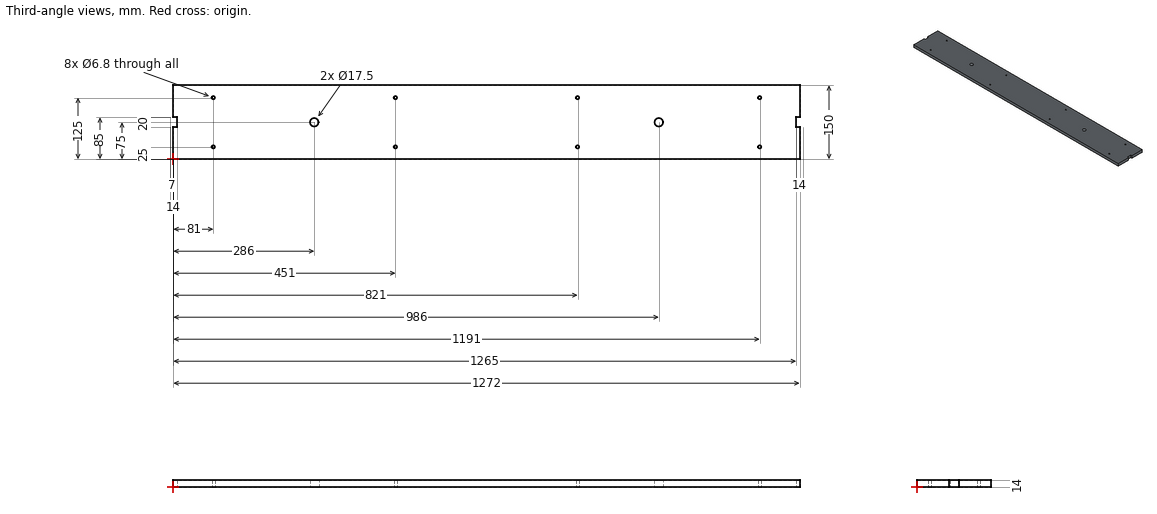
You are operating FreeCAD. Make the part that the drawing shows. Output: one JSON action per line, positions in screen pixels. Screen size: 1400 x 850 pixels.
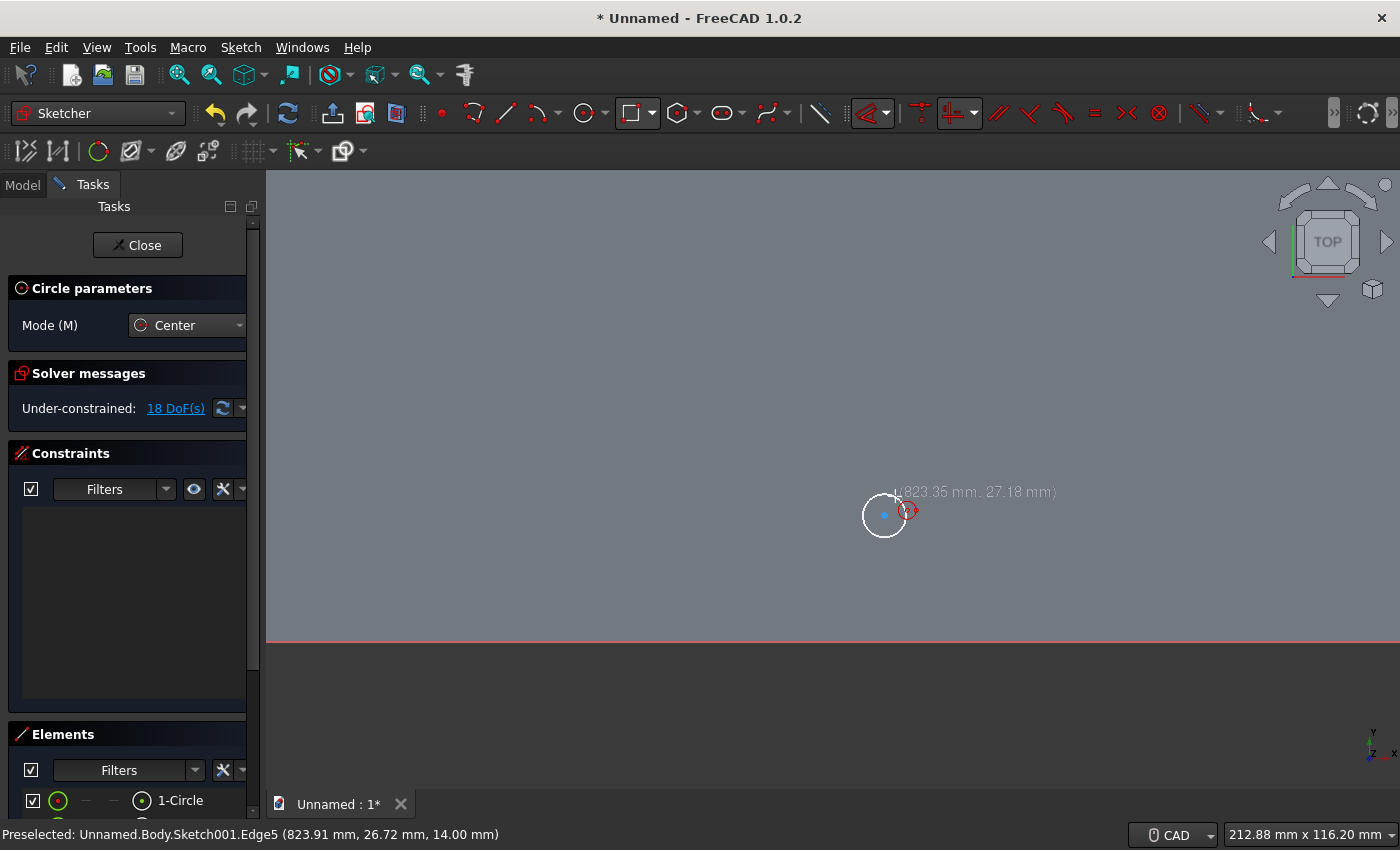
{"action": "scroll", "coordinate": [898, 502], "scroll_direction": "down", "scroll_amount": 11}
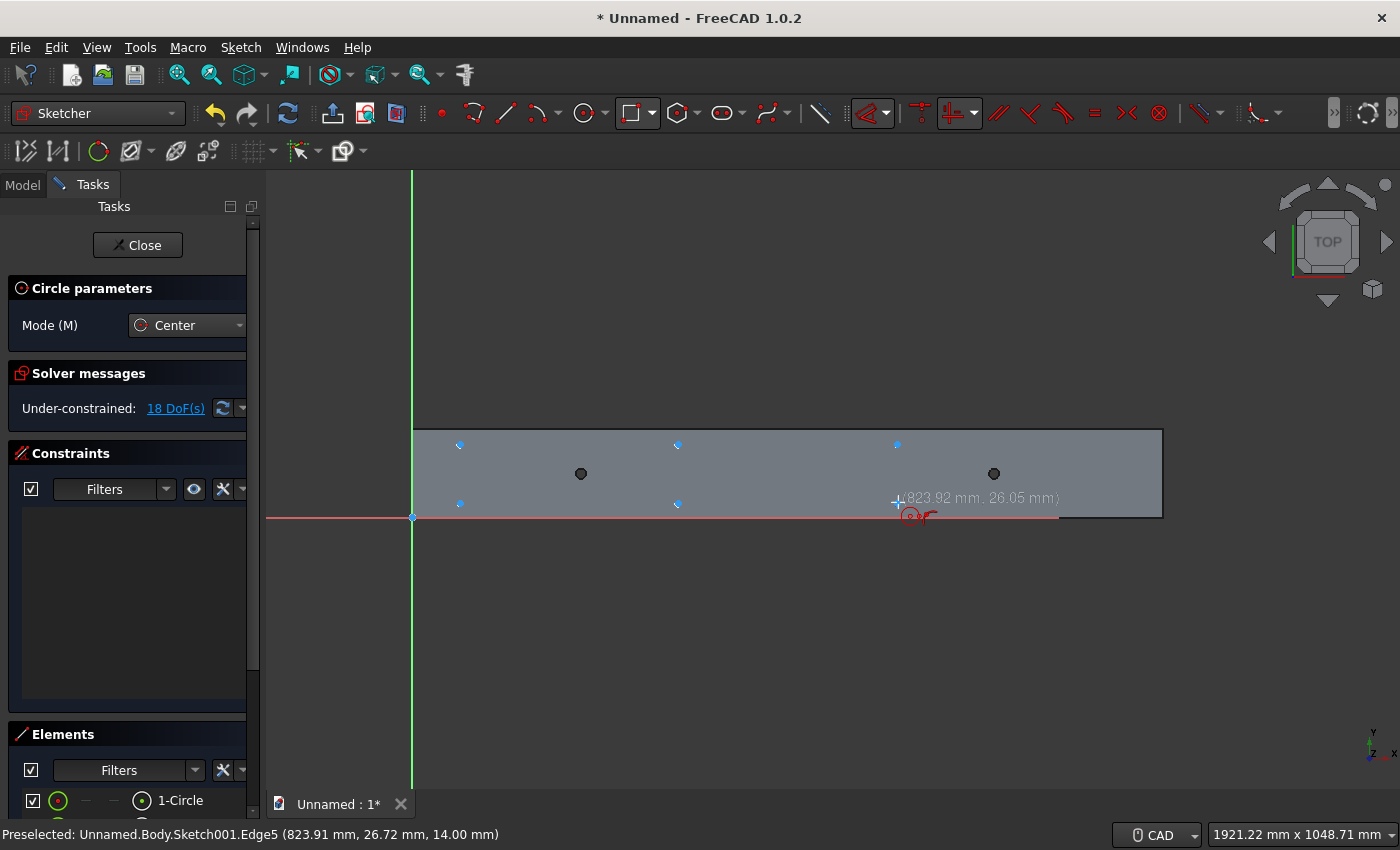
{"action": "scroll", "coordinate": [1115, 444], "scroll_direction": "up", "scroll_amount": 13}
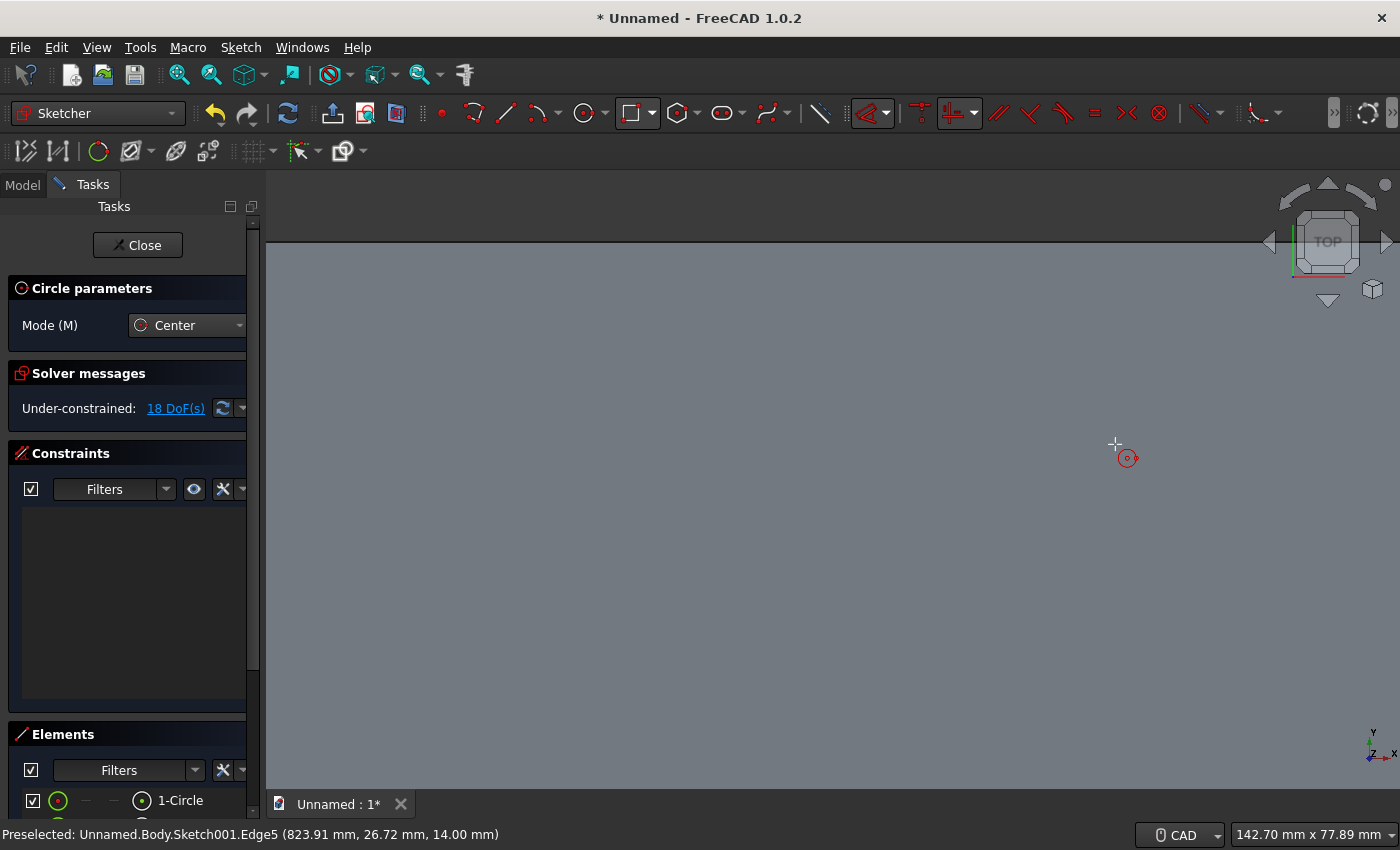
{"action": "scroll", "coordinate": [1116, 444], "scroll_direction": "down", "scroll_amount": 13}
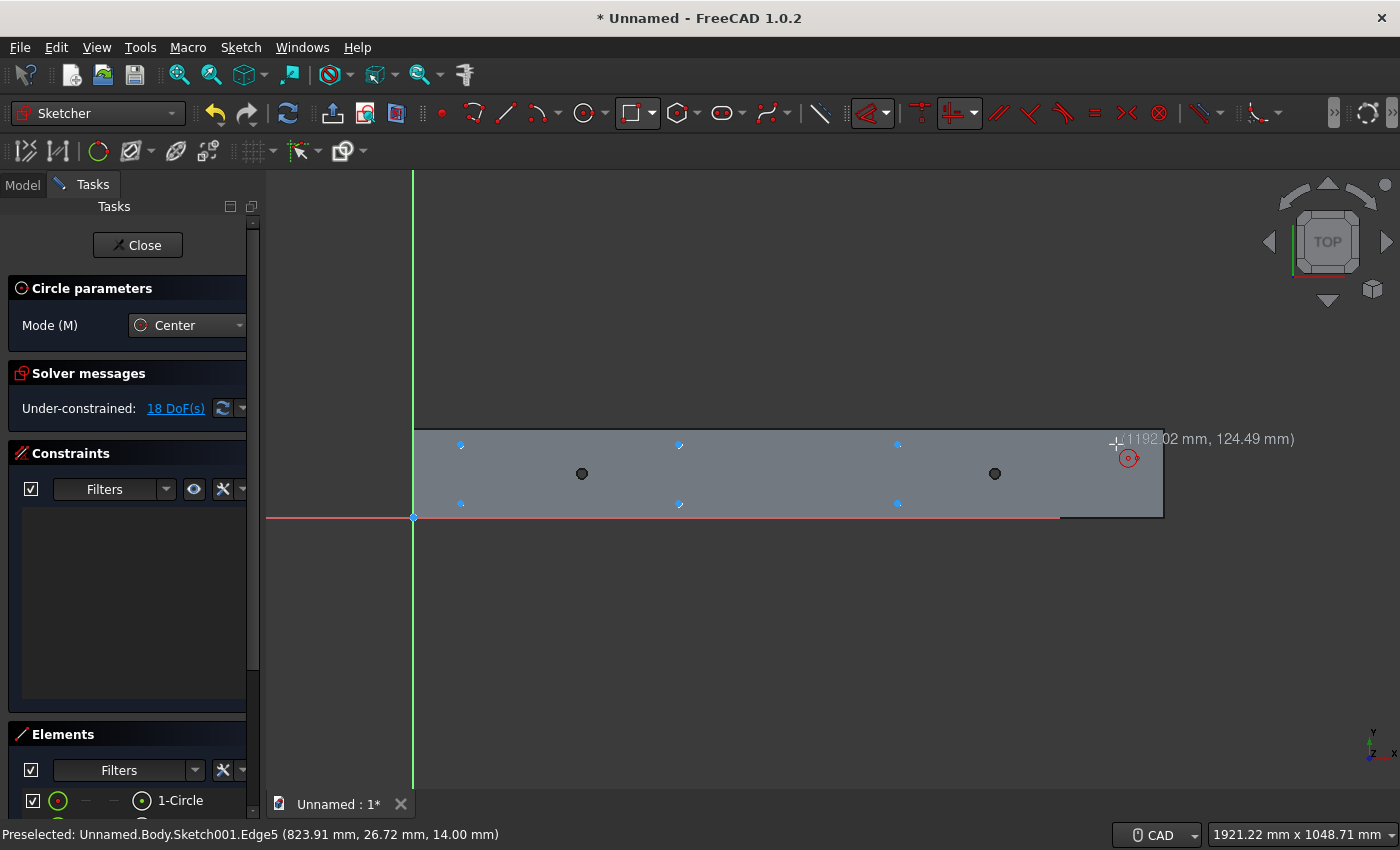
{"action": "left_click", "coordinate": [1116, 444]}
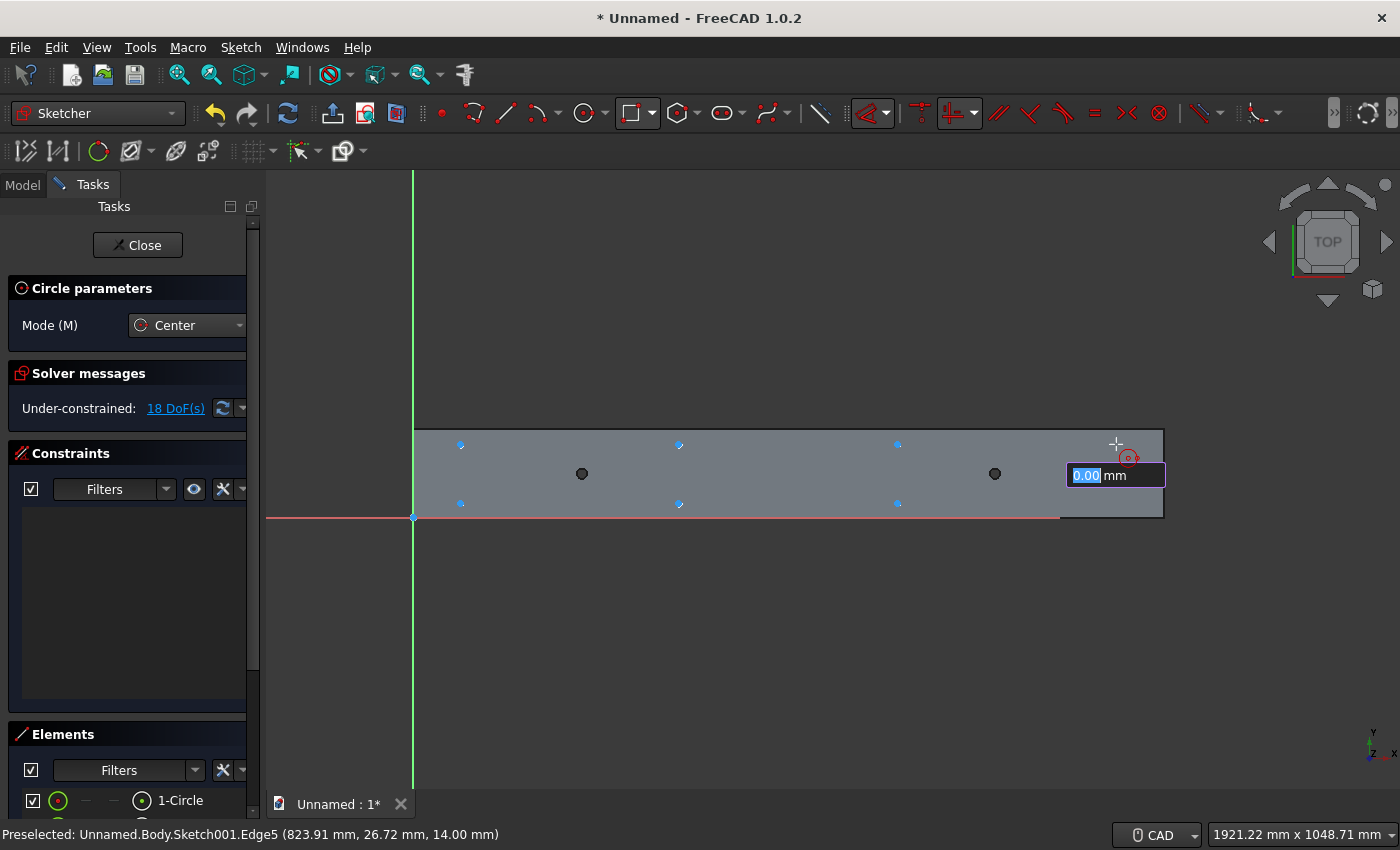
{"action": "scroll", "coordinate": [1118, 443], "scroll_direction": "up", "scroll_amount": 11}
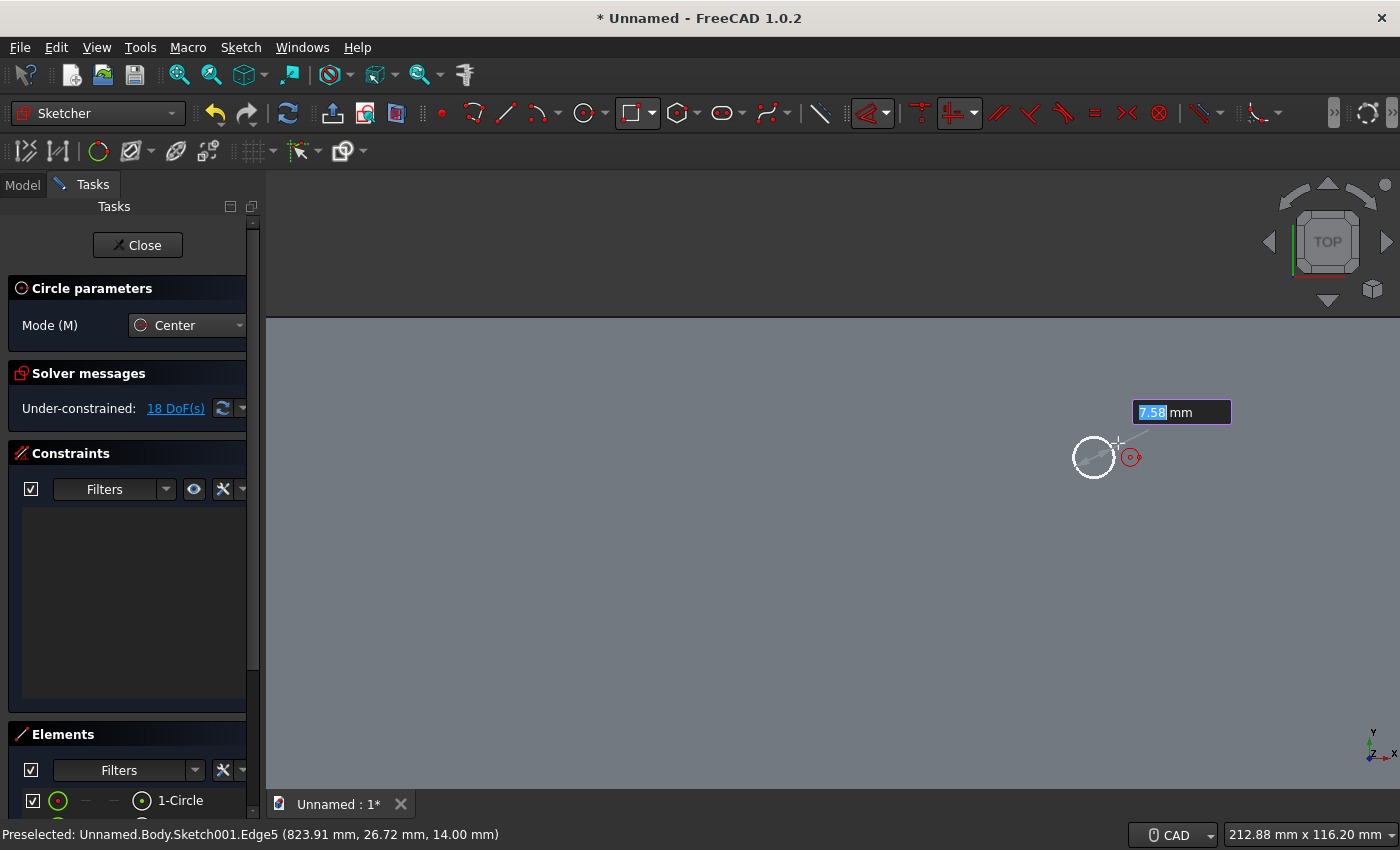
{"action": "left_click", "coordinate": [1108, 437]}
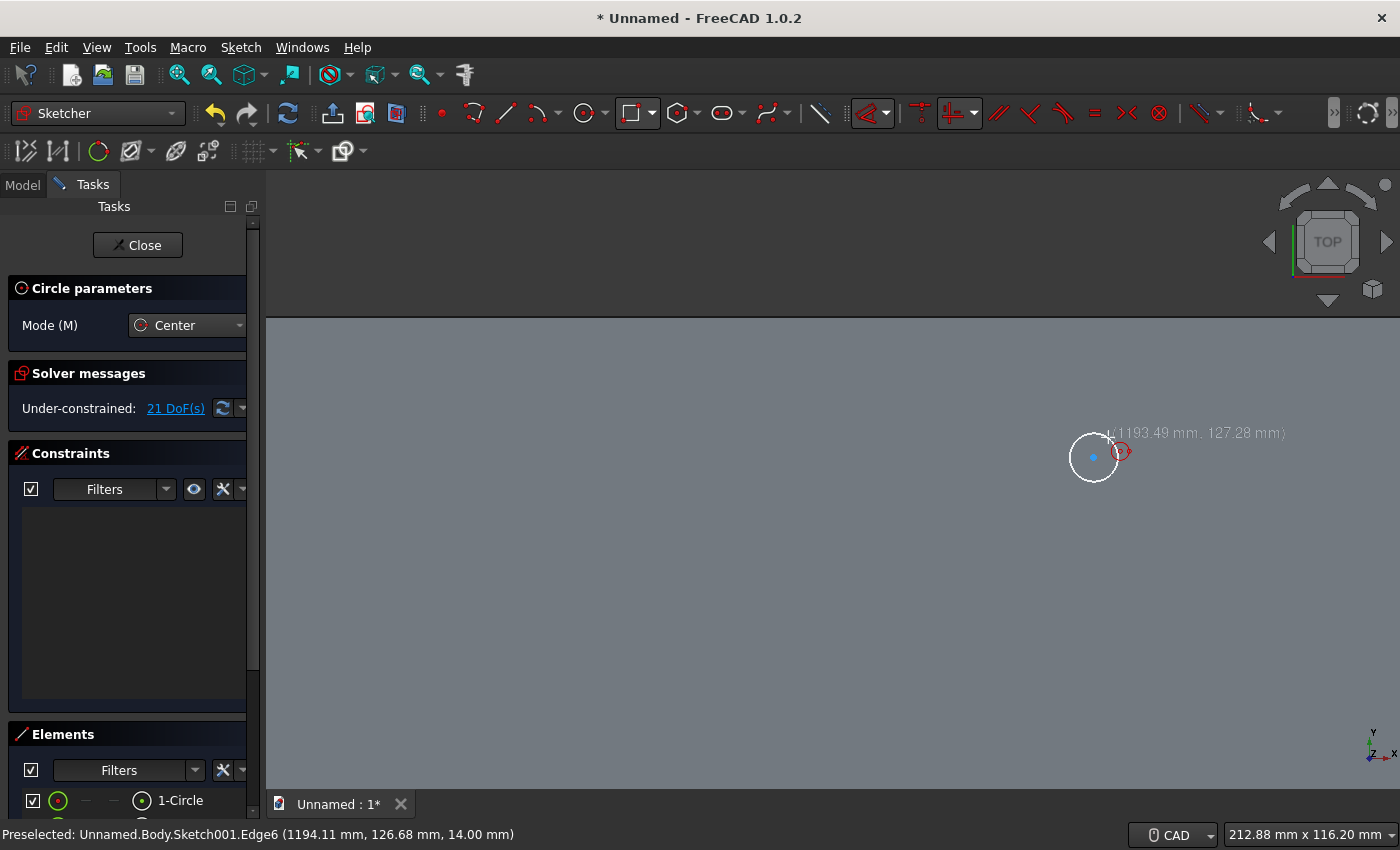
{"action": "scroll", "coordinate": [1118, 443], "scroll_direction": "down", "scroll_amount": 11}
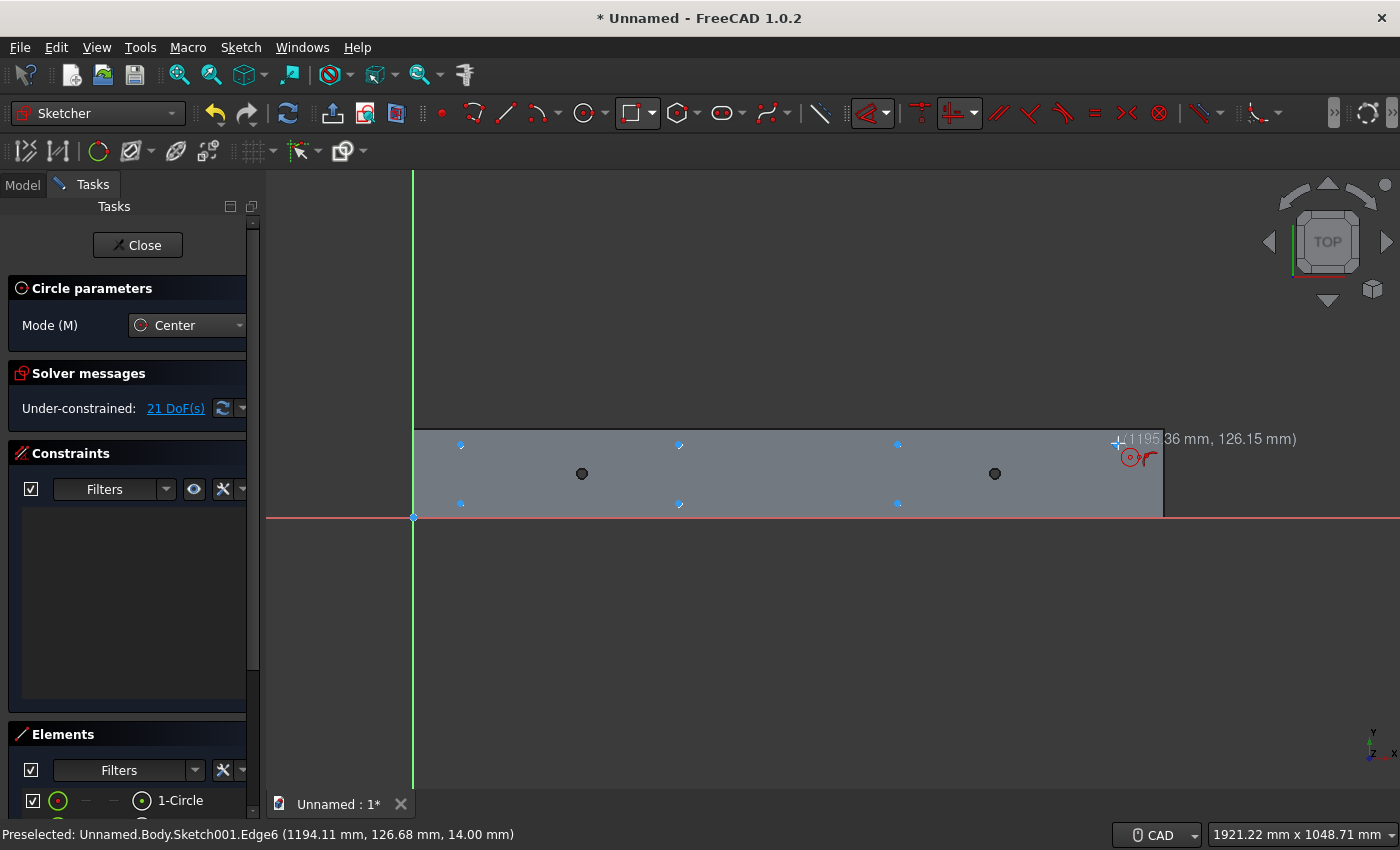
{"action": "scroll", "coordinate": [1116, 503], "scroll_direction": "up", "scroll_amount": 13}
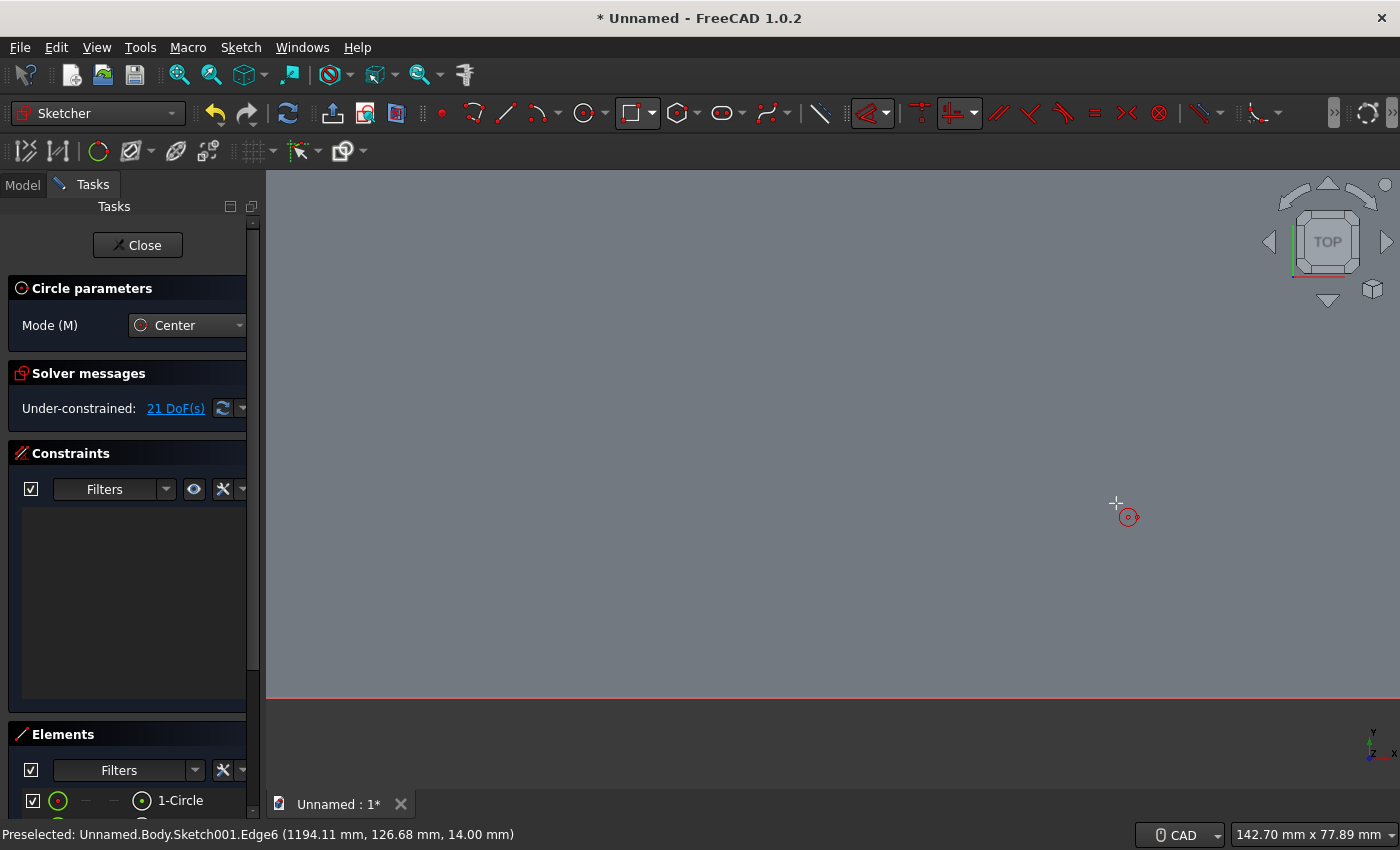
{"action": "scroll", "coordinate": [1116, 503], "scroll_direction": "down", "scroll_amount": 13}